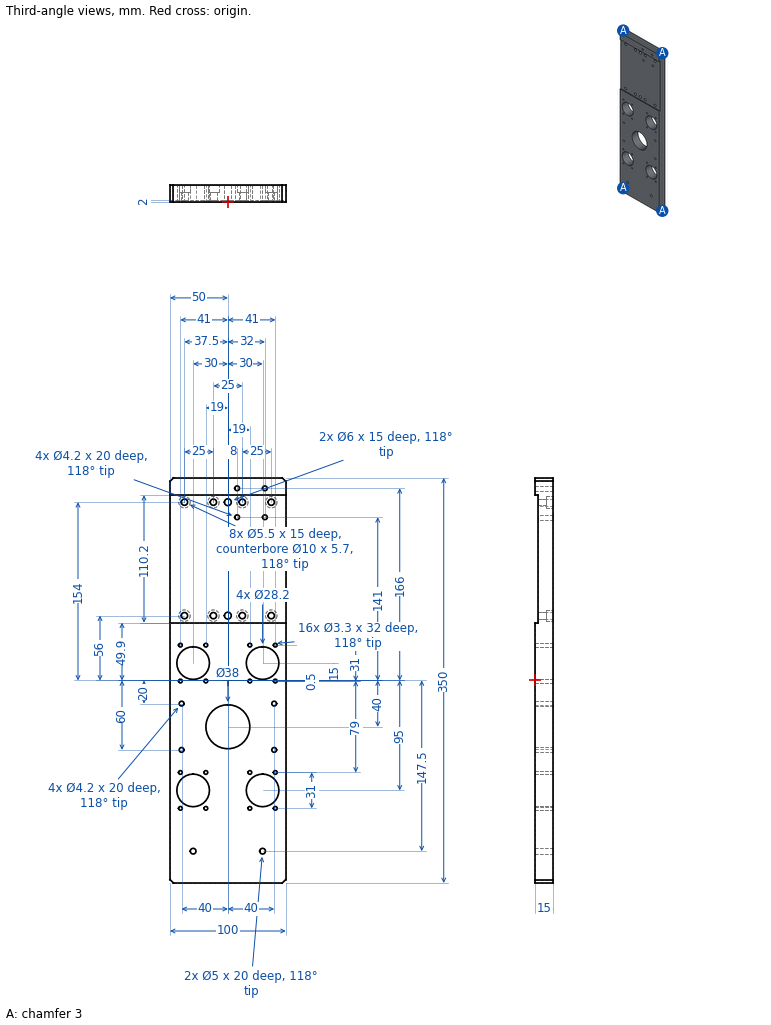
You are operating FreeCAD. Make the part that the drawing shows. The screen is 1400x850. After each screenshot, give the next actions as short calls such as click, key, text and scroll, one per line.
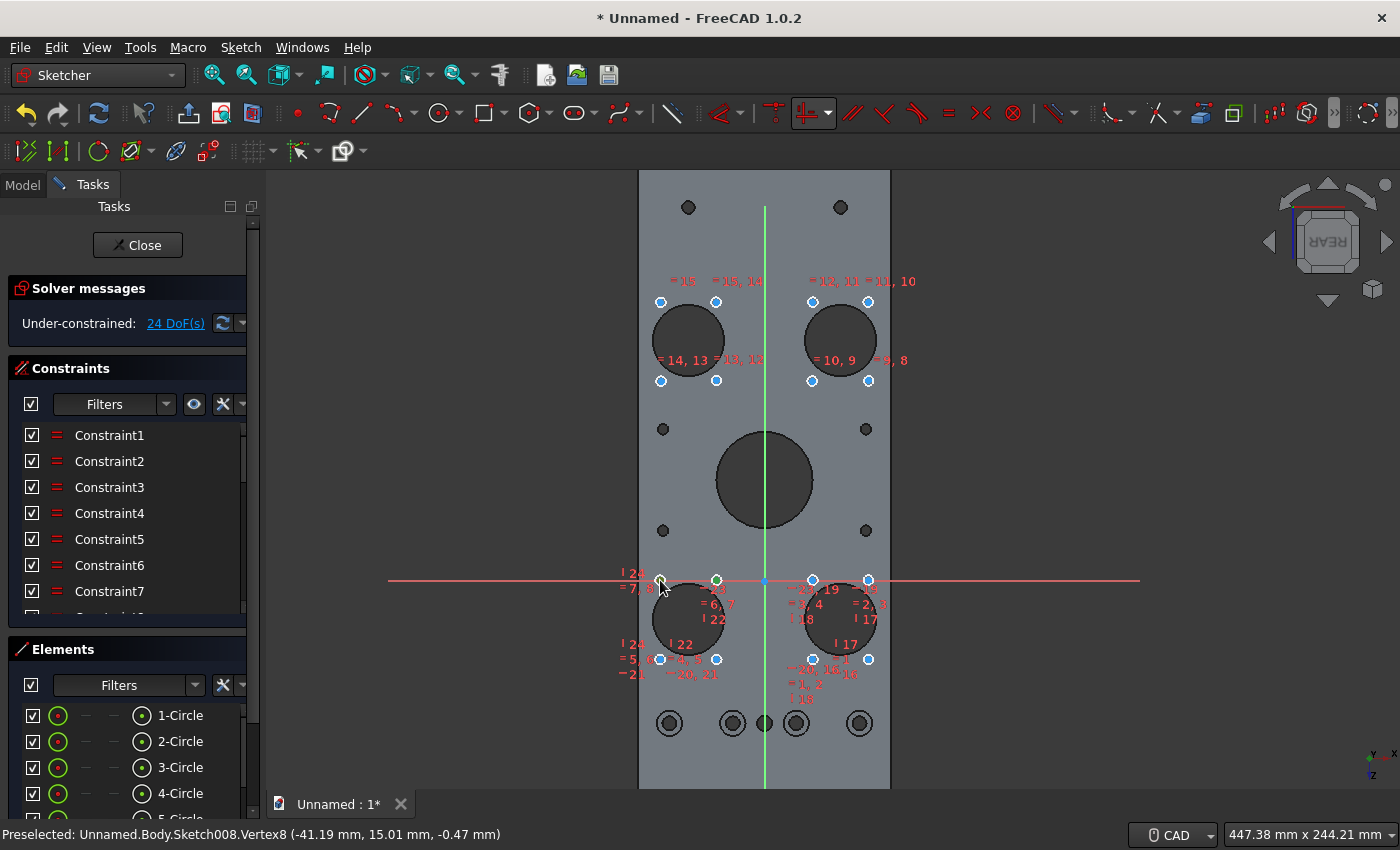
key(h)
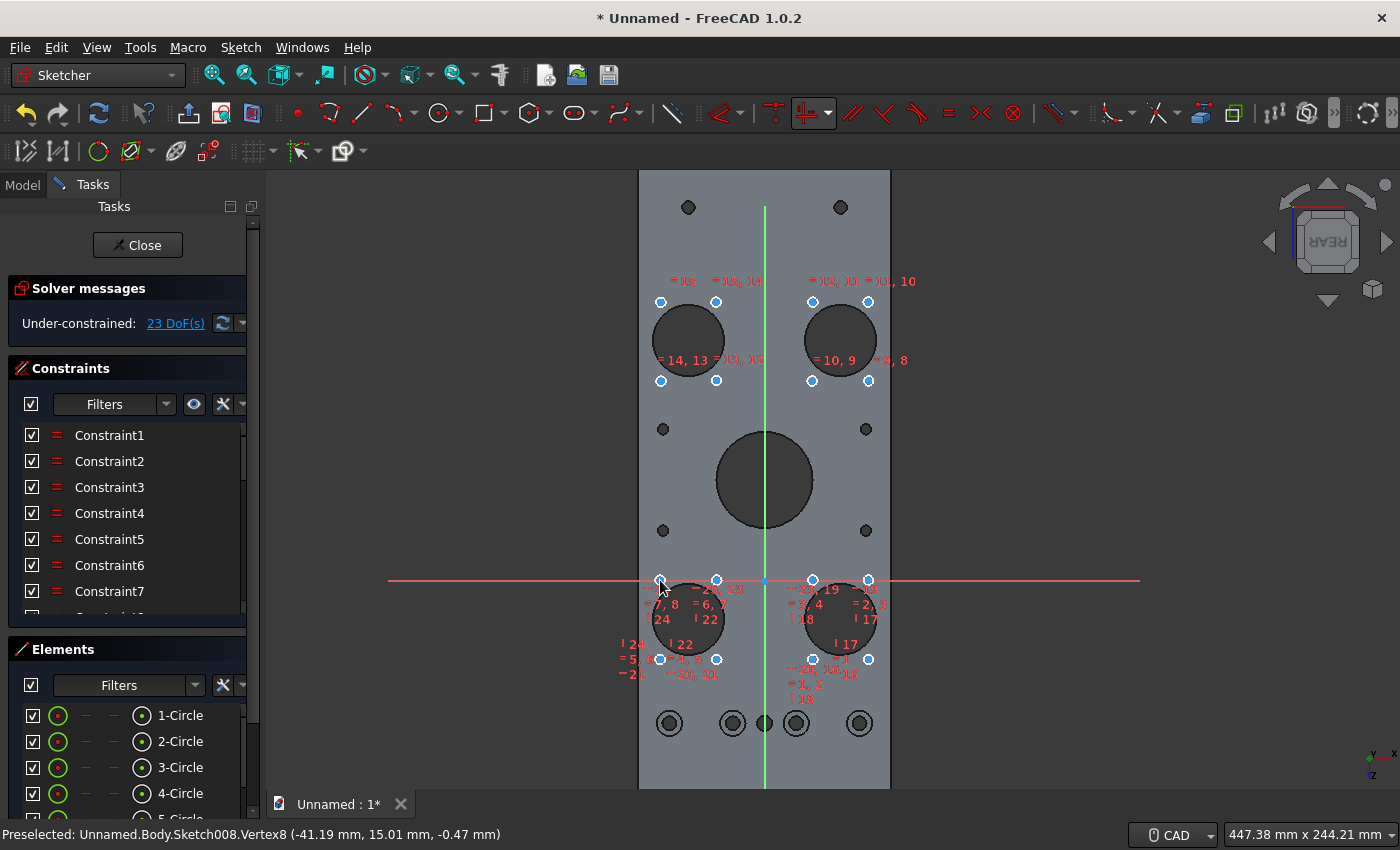
click(868, 580)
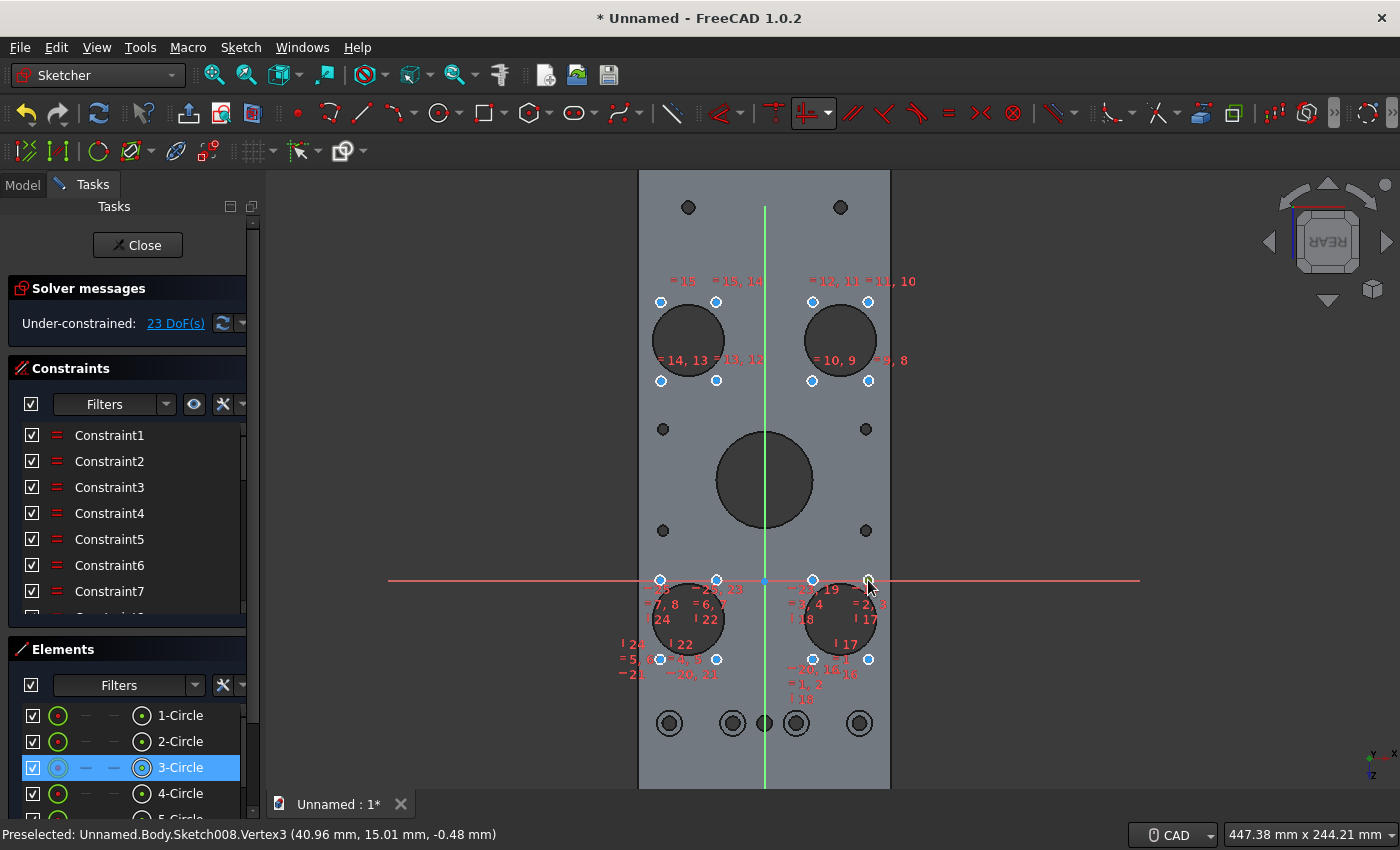
click(869, 381)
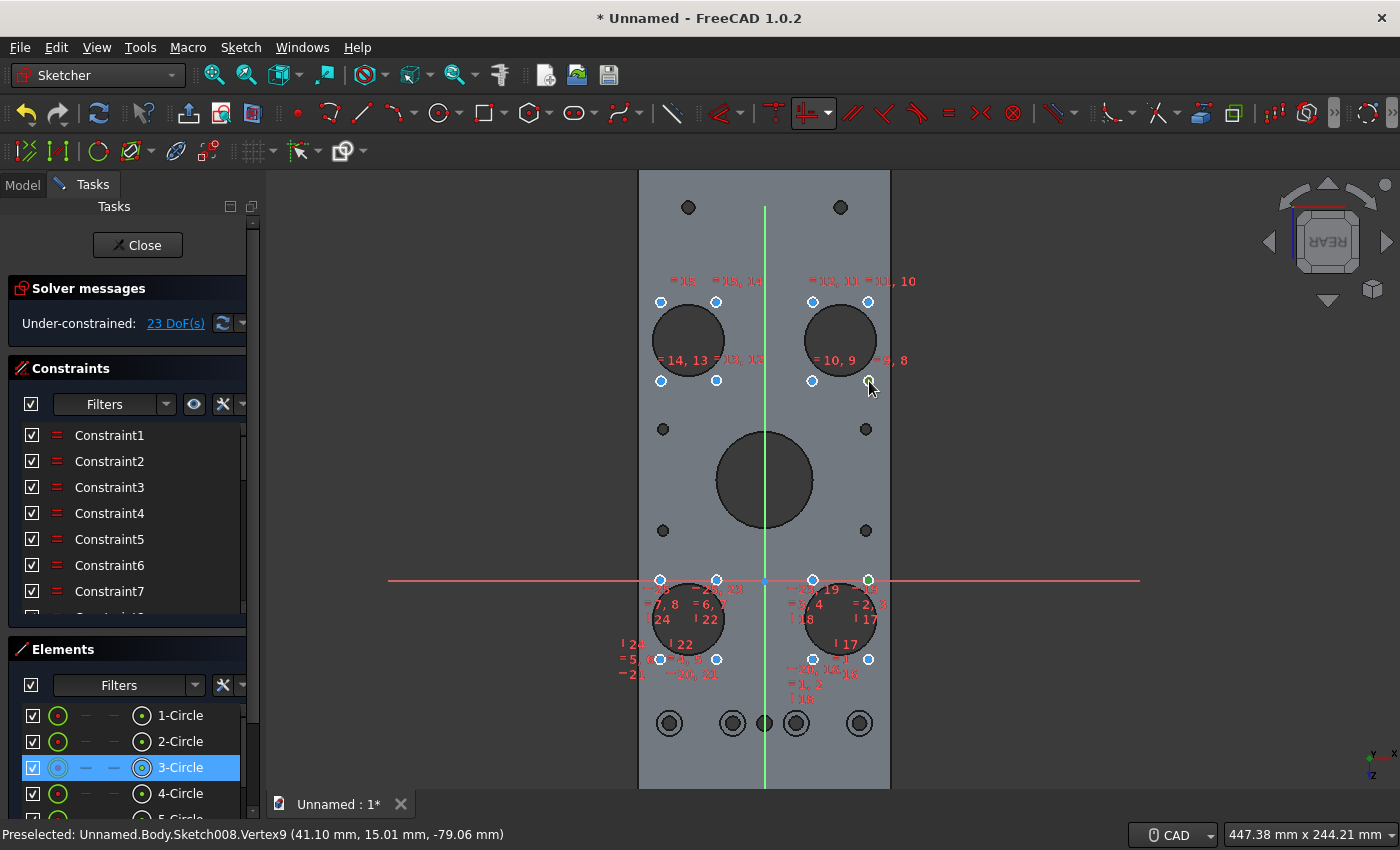
key(v)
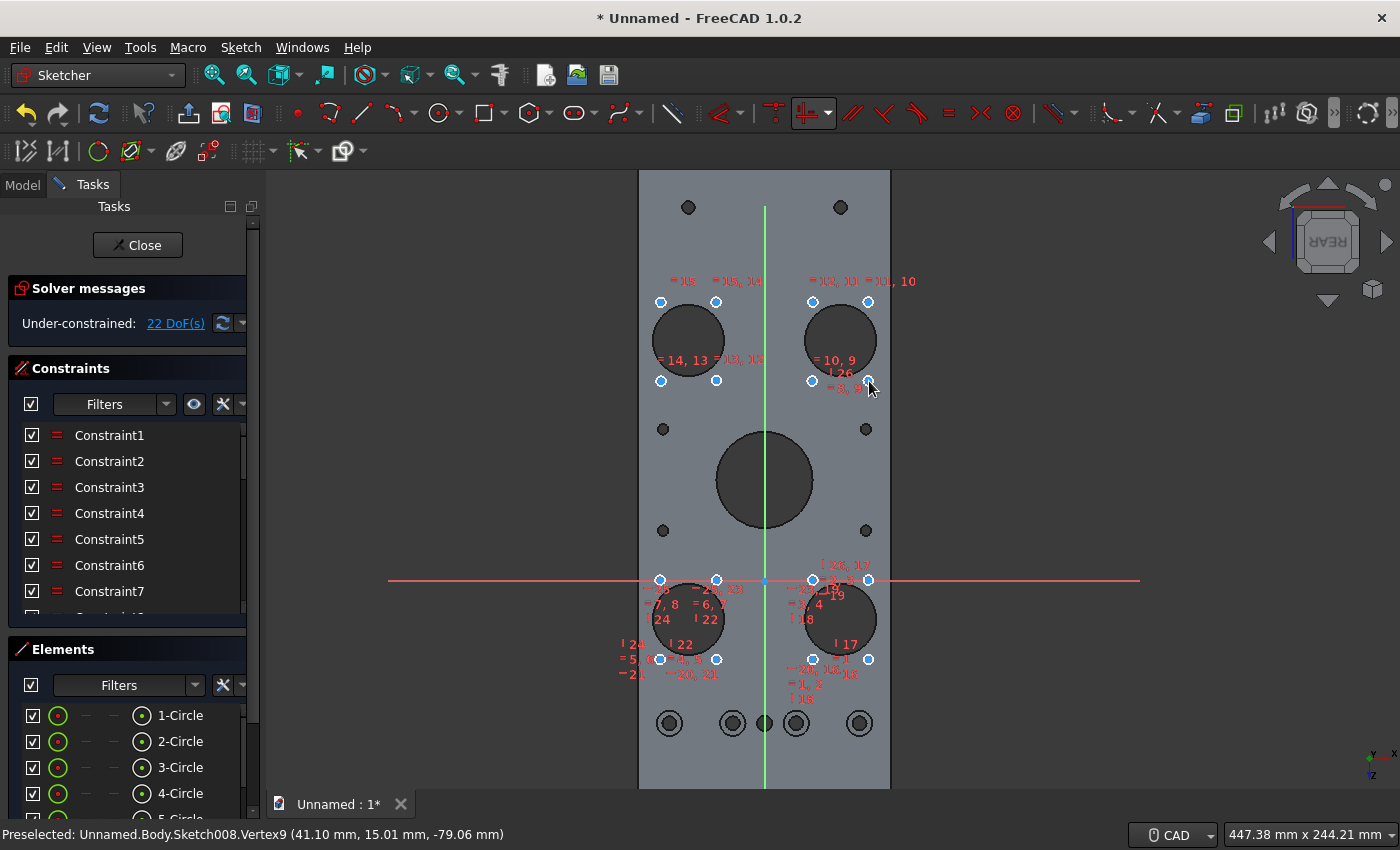
click(813, 580)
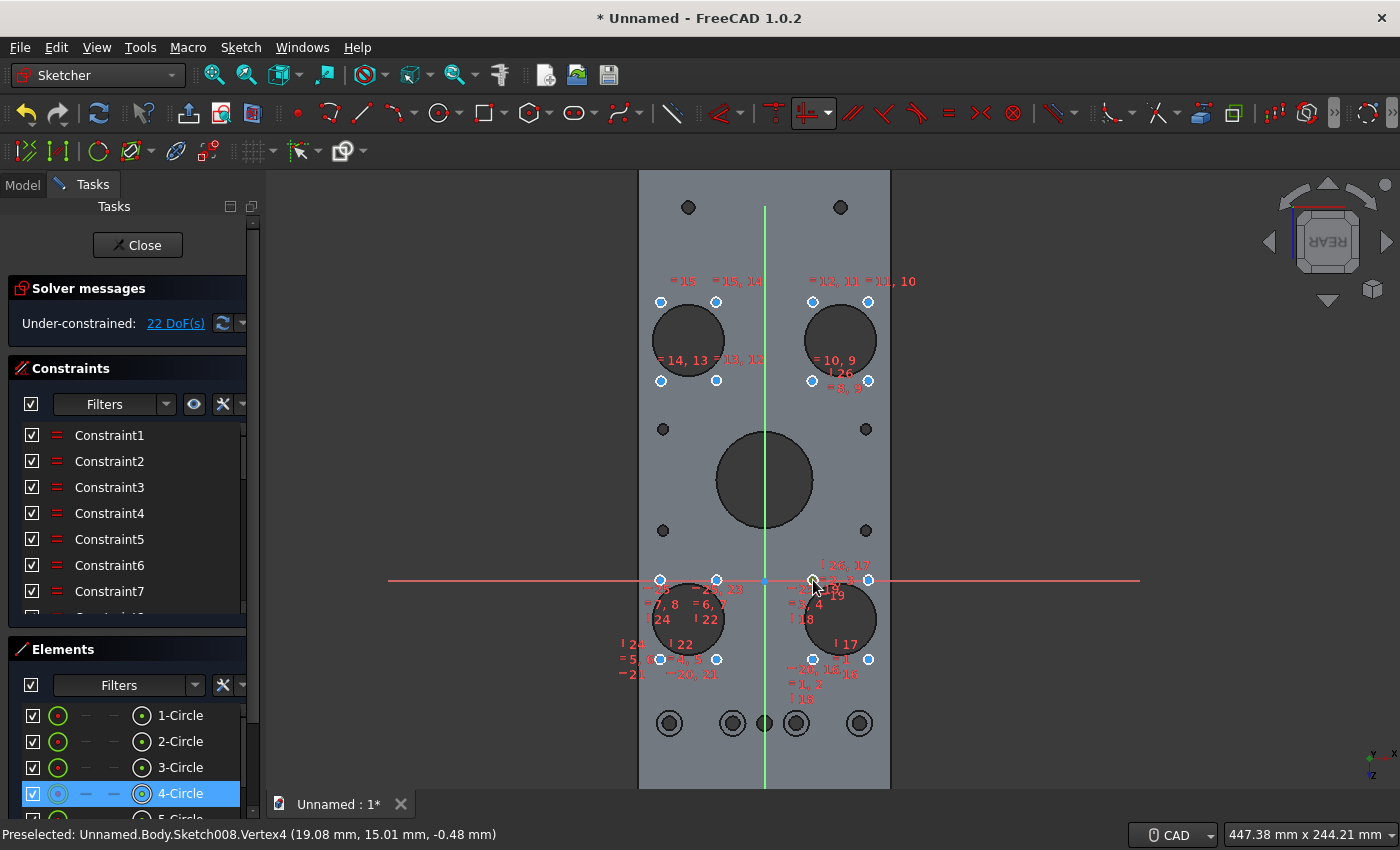
click(812, 381)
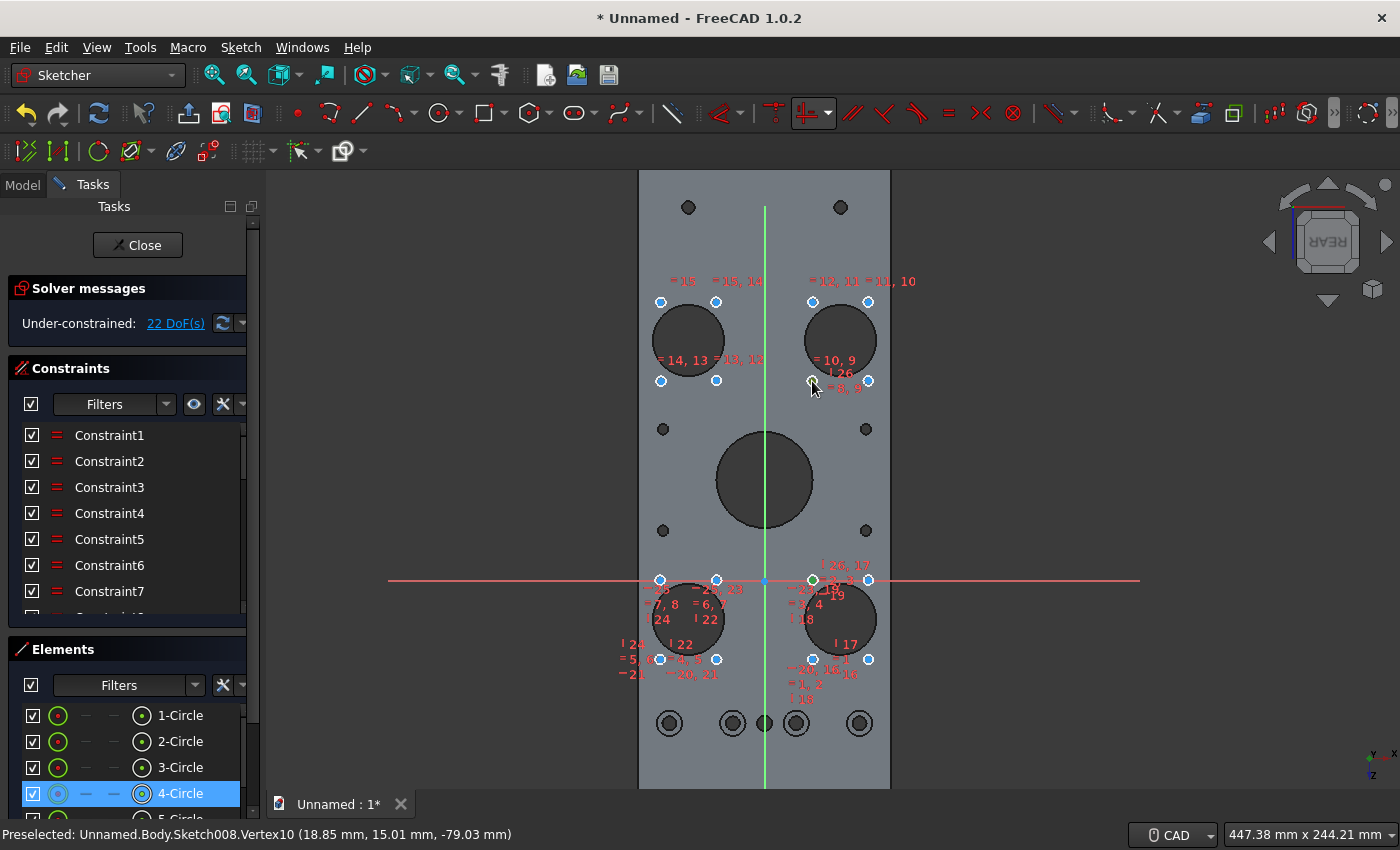
key(v)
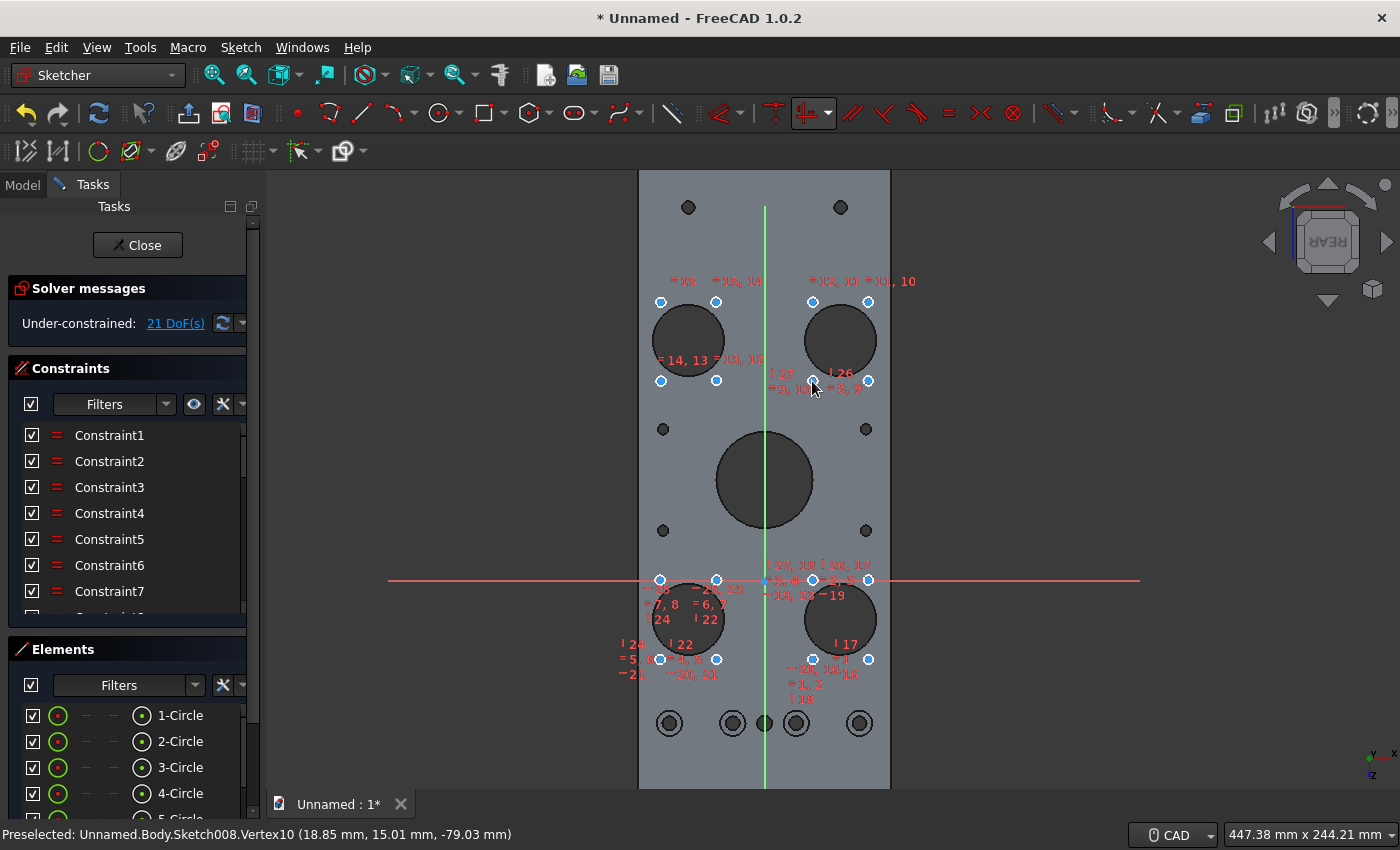
click(868, 381)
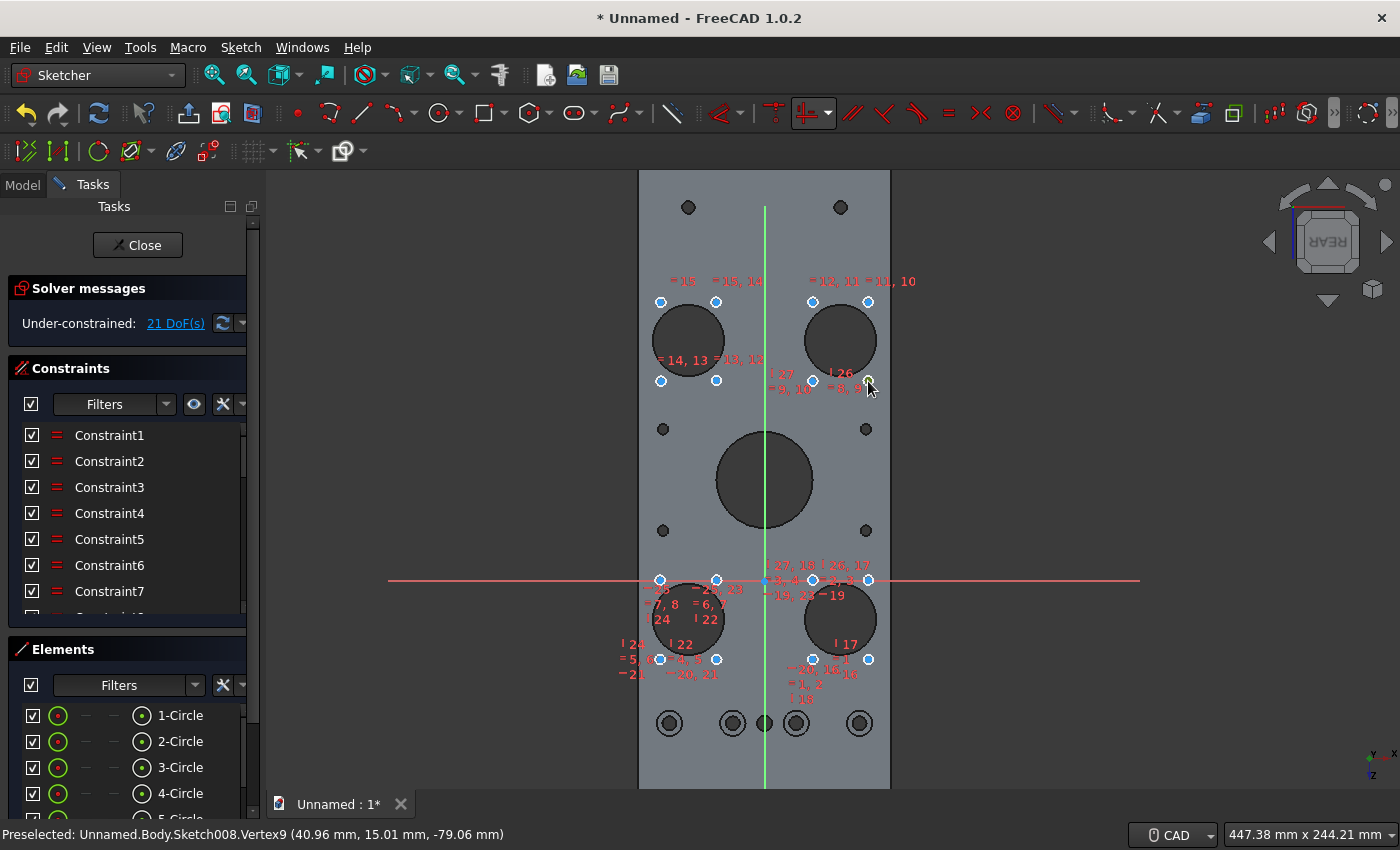
click(813, 381)